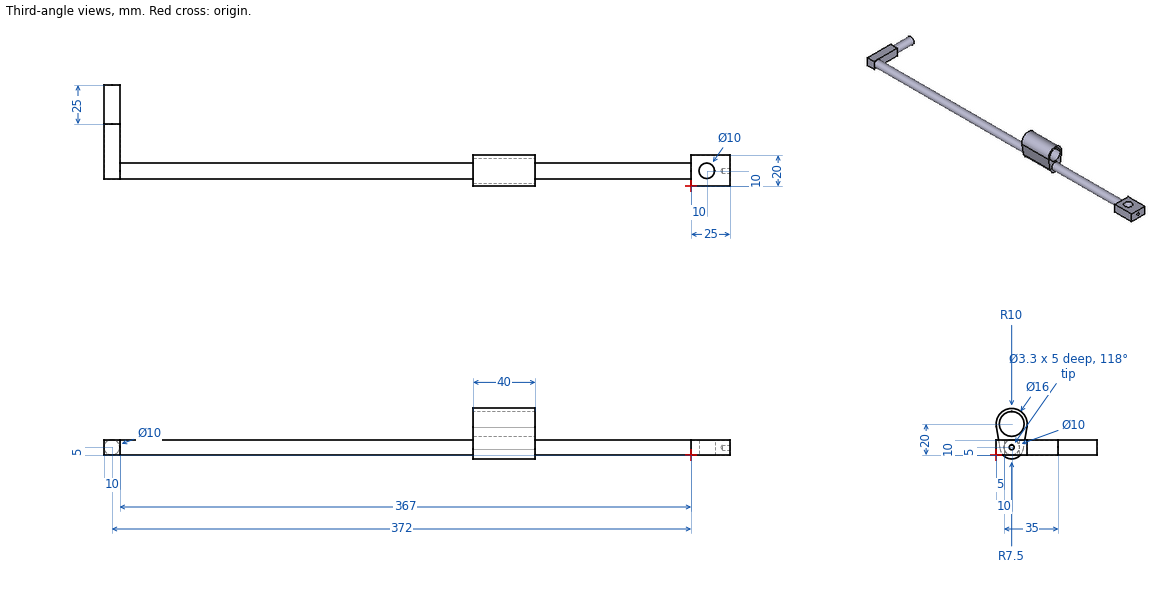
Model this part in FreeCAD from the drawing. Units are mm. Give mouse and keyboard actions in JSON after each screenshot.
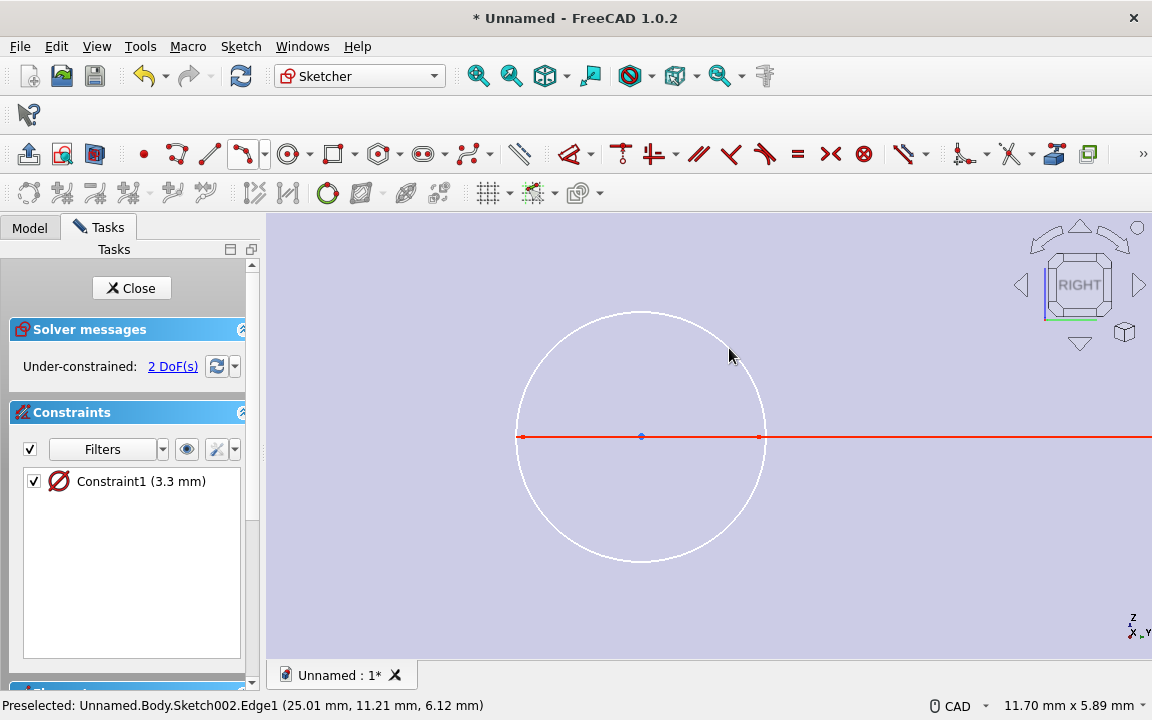
{"action": "key", "text": "d"}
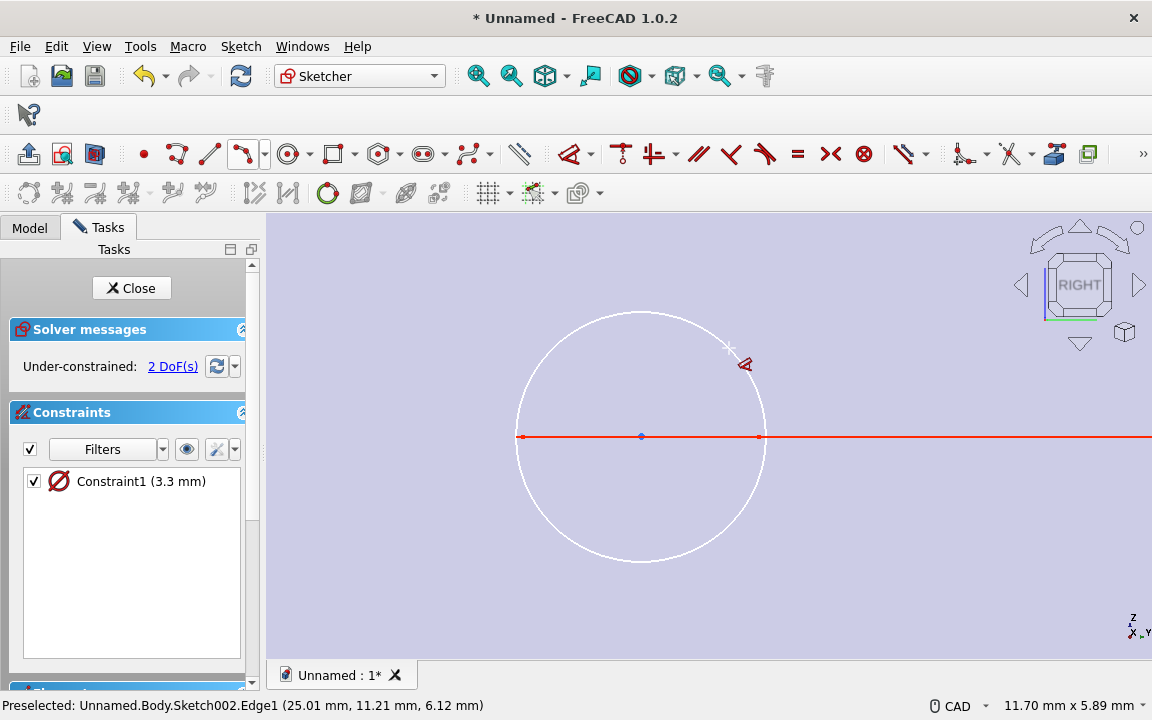
{"action": "left_click", "coordinate": [641, 437]}
{"action": "left_click", "coordinate": [675, 534]}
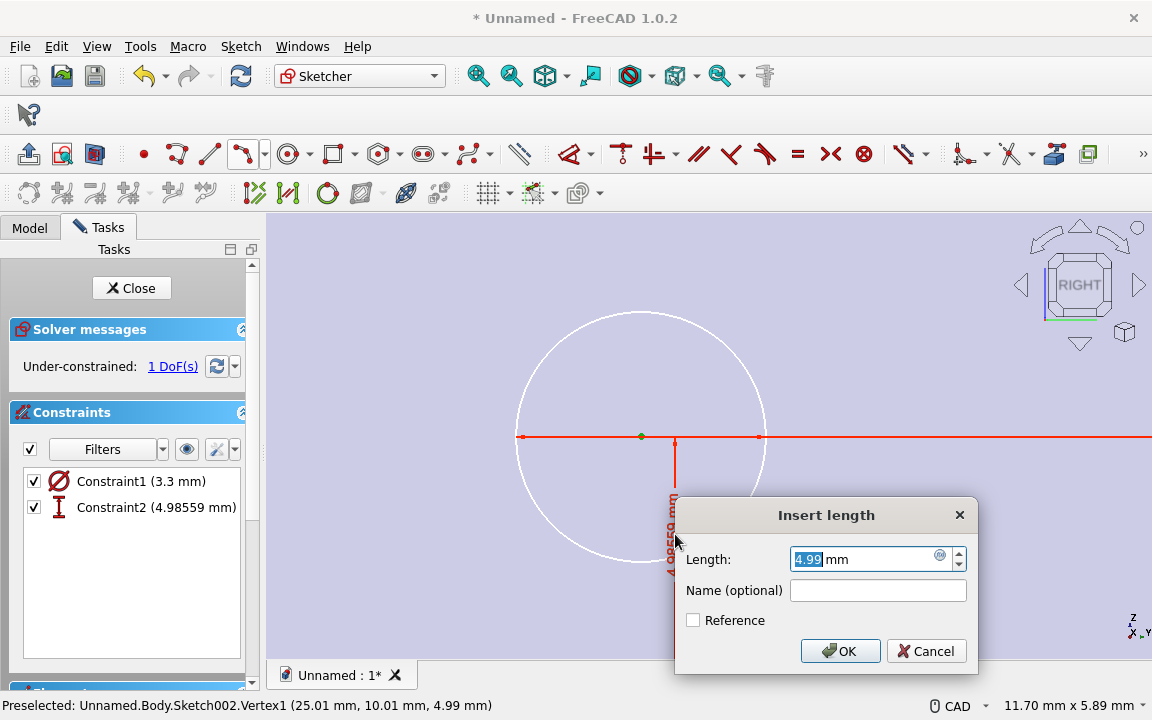
{"action": "type", "text": "5"}
{"action": "key", "text": "Return"}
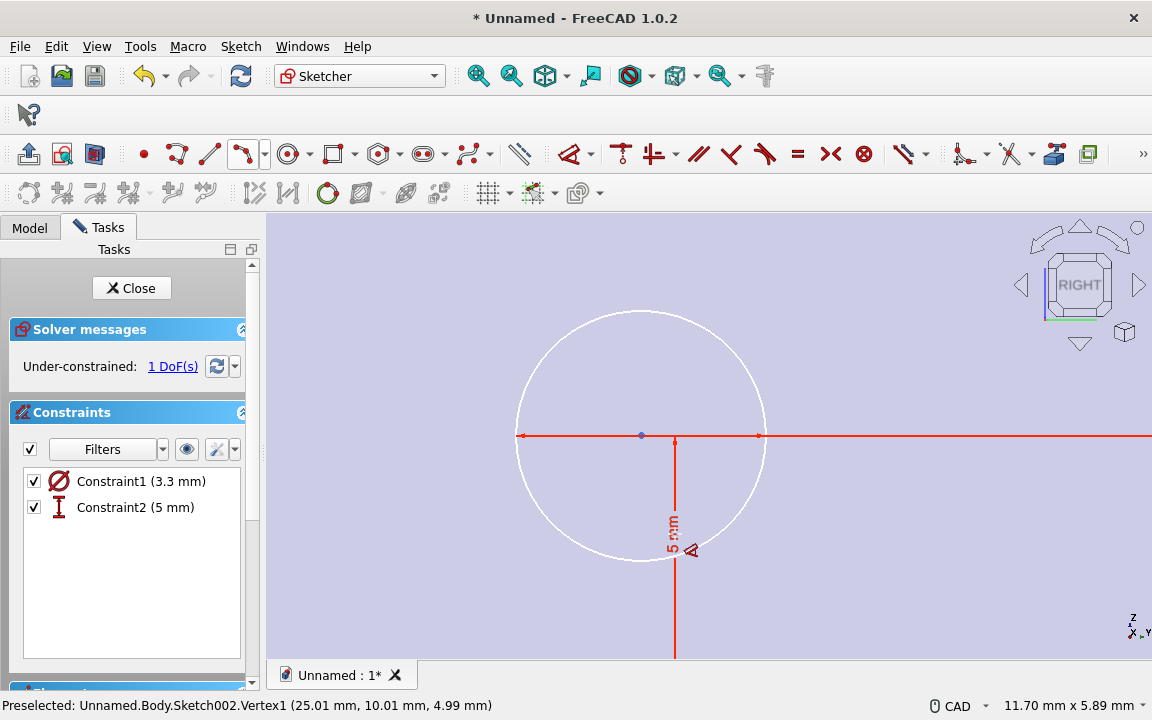
{"action": "left_click", "coordinate": [641, 436]}
{"action": "left_click", "coordinate": [467, 402]}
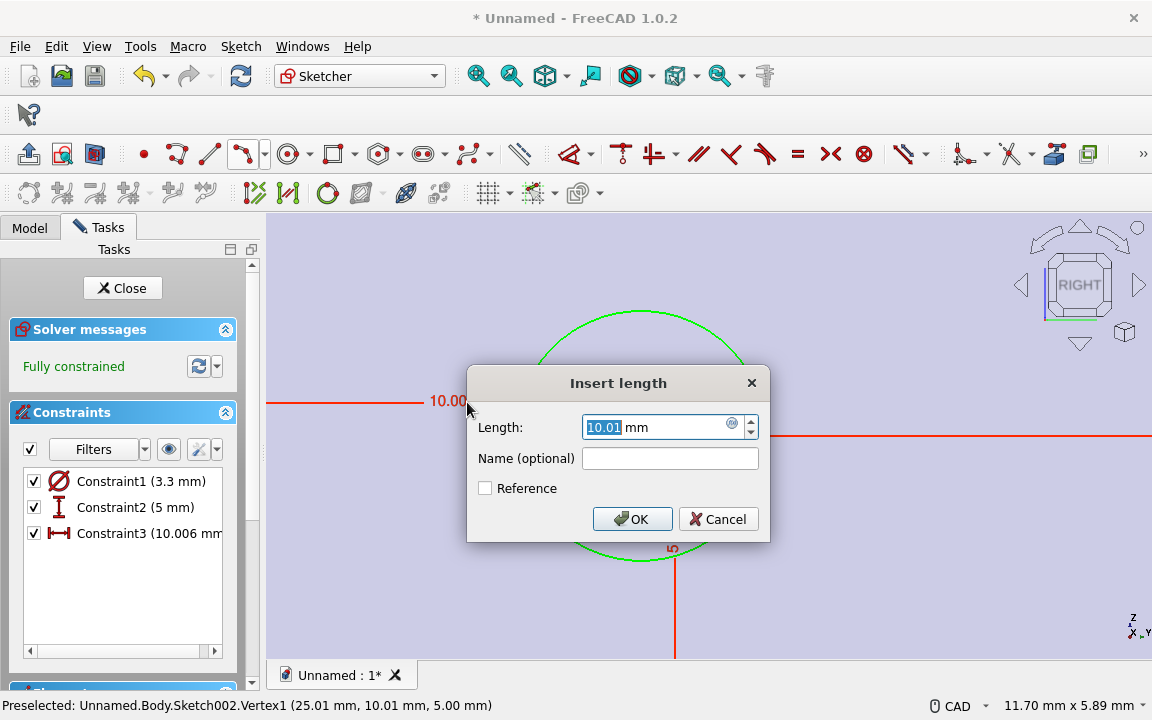
{"action": "type", "text": "10"}
{"action": "key", "text": "Return"}
{"action": "key", "text": "Escape"}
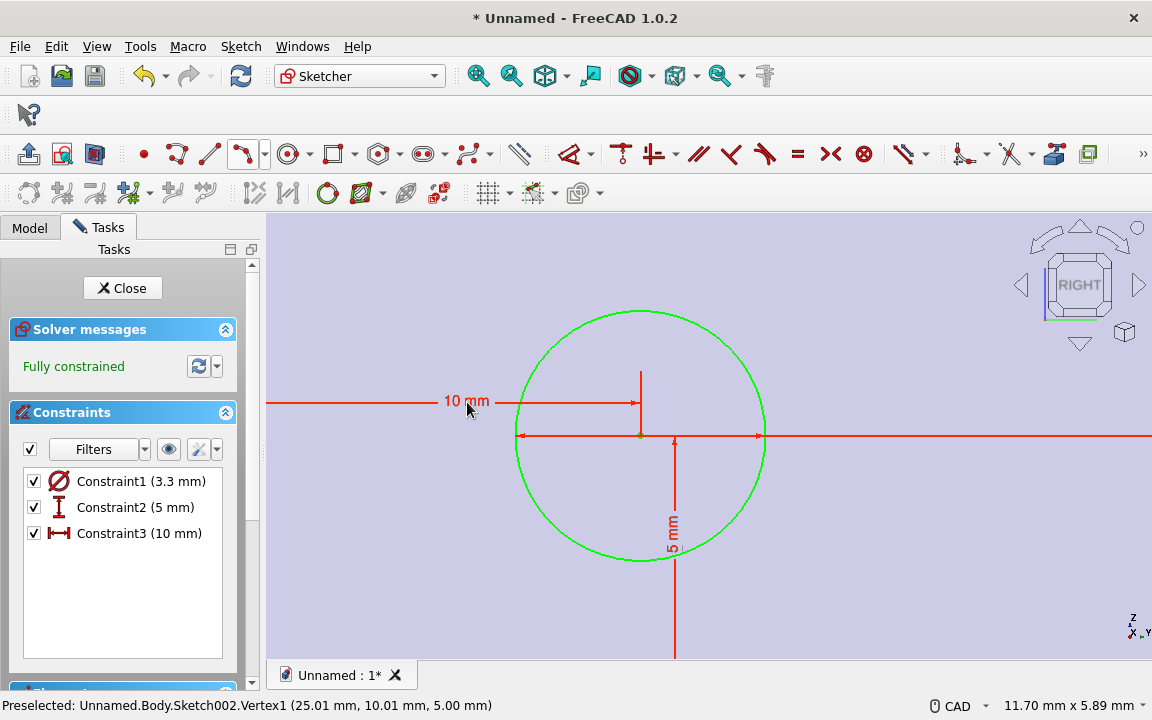
{"action": "left_click", "coordinate": [123, 288]}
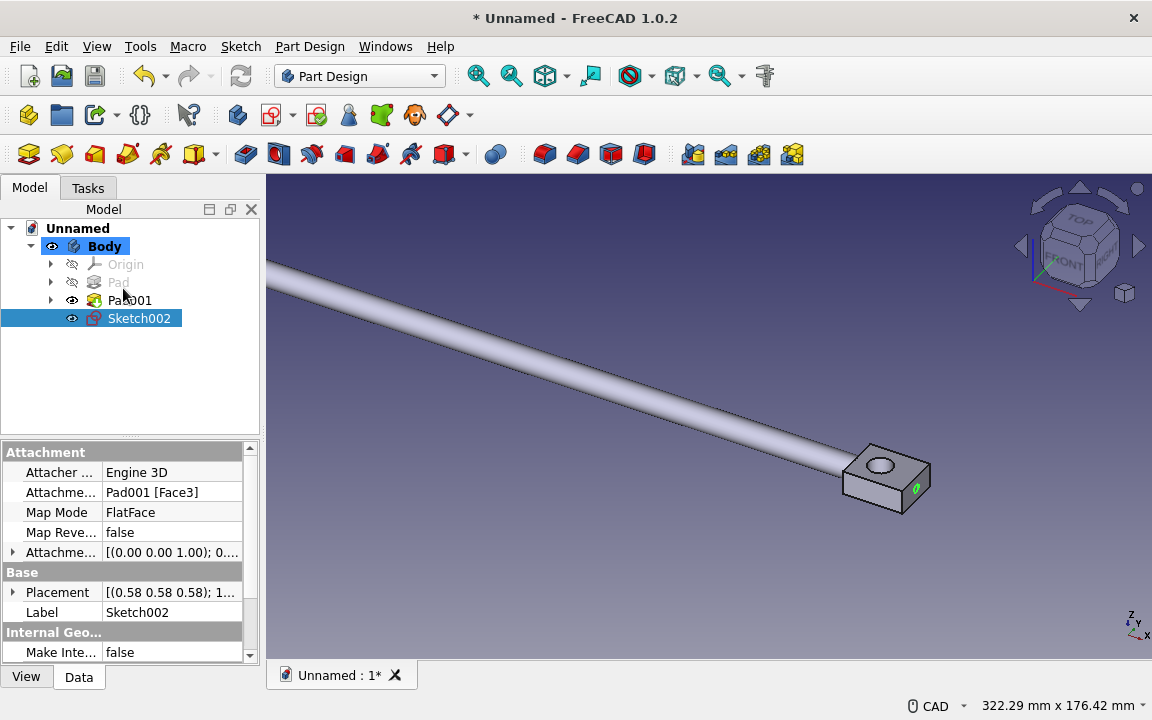
{"action": "left_click", "coordinate": [279, 154]}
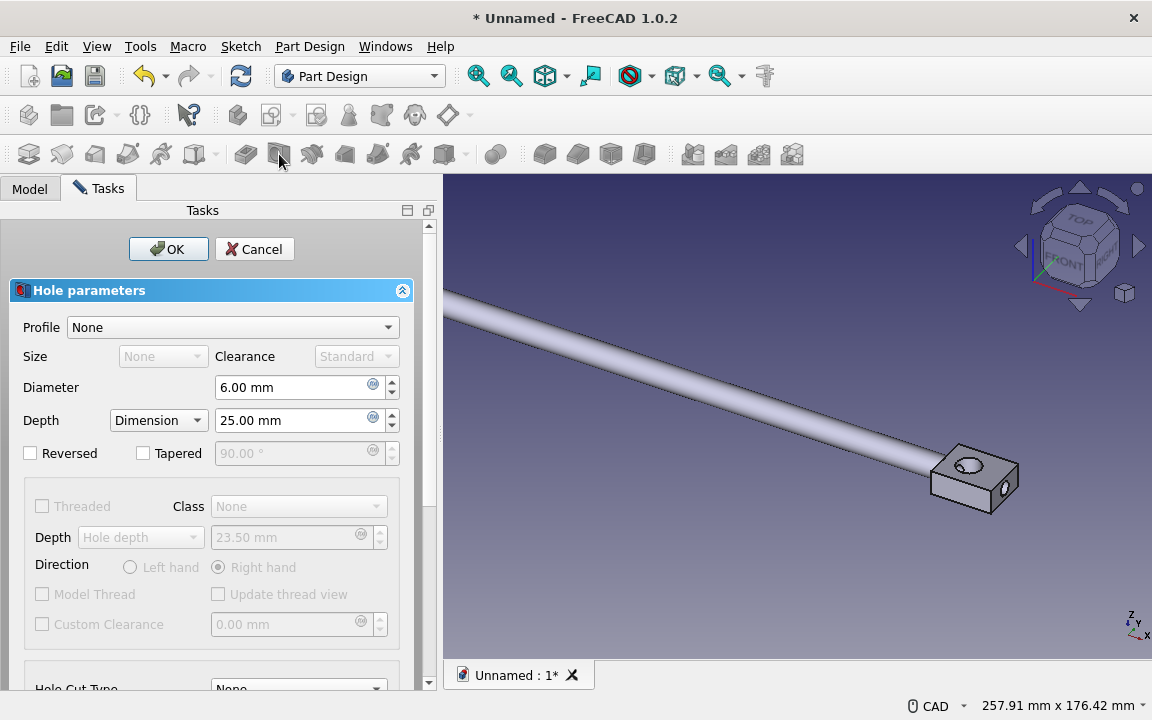
{"action": "triple_click", "coordinate": [300, 388]}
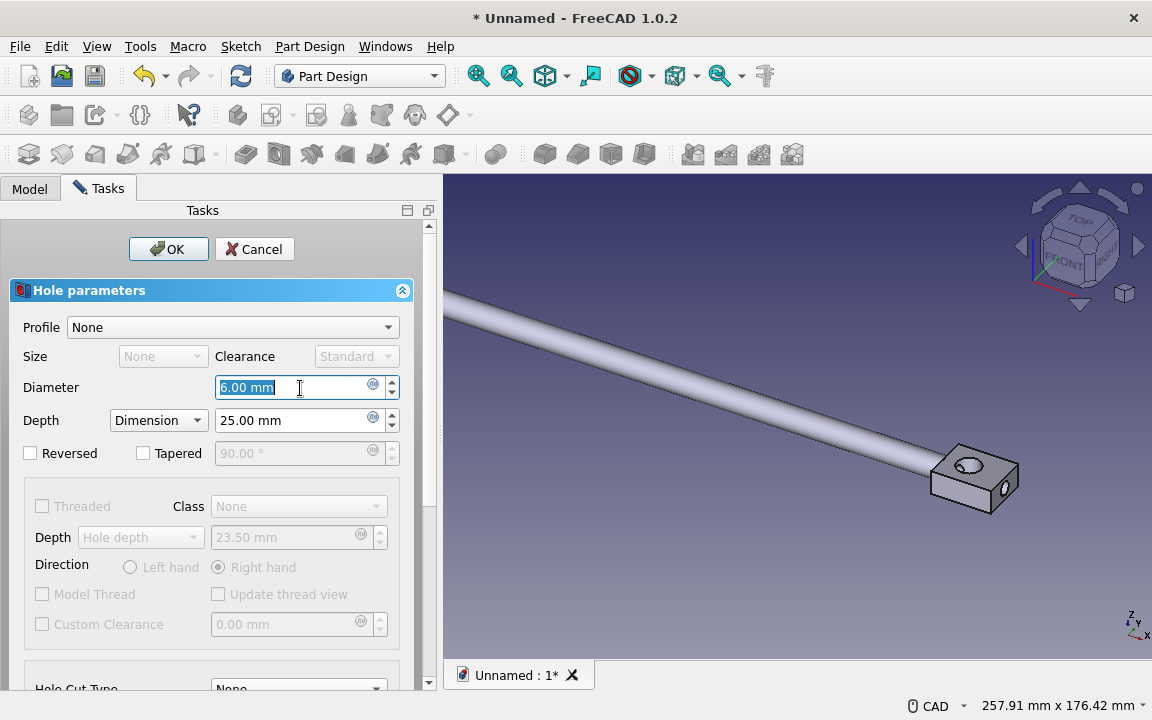
{"action": "type", "text": "3.3"}
{"action": "key", "text": "Tab"}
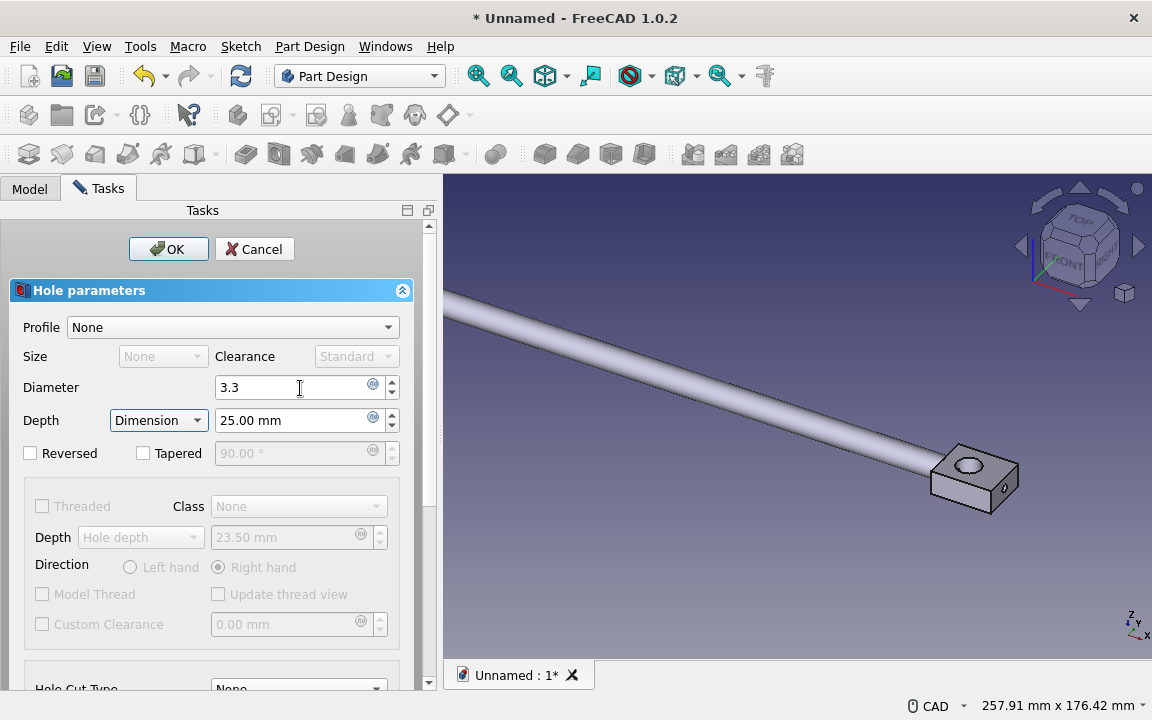
{"action": "triple_click", "coordinate": [300, 420]}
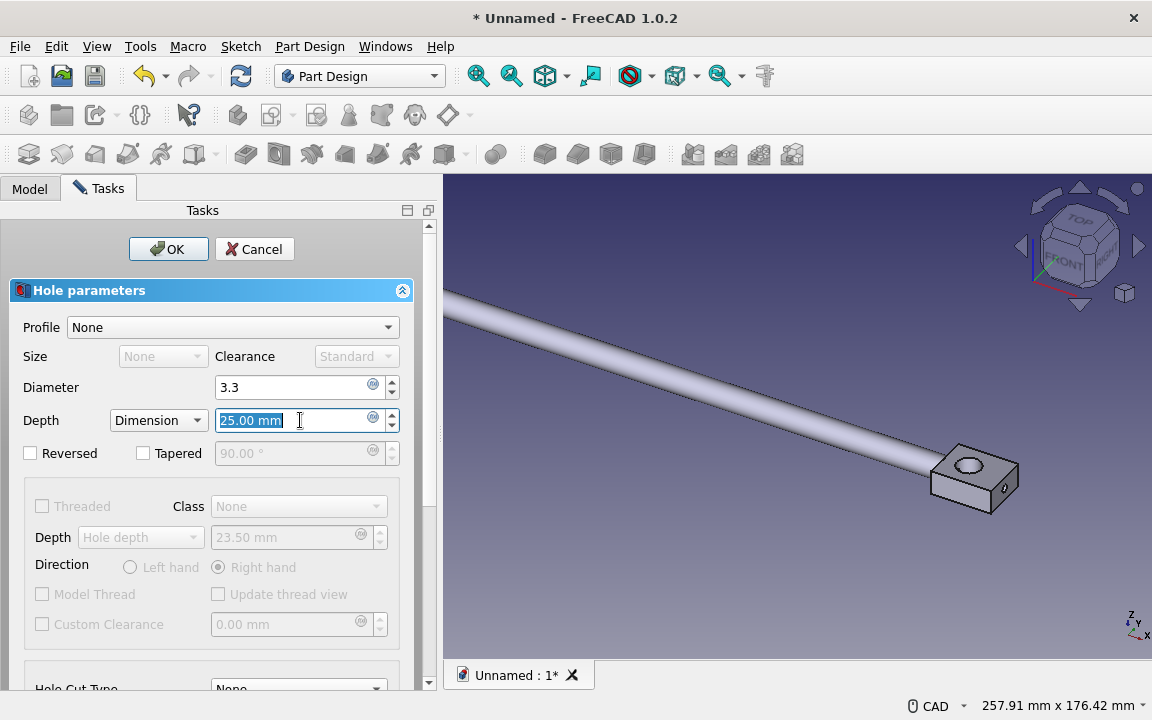
{"action": "type", "text": "5"}
{"action": "key", "text": "Tab"}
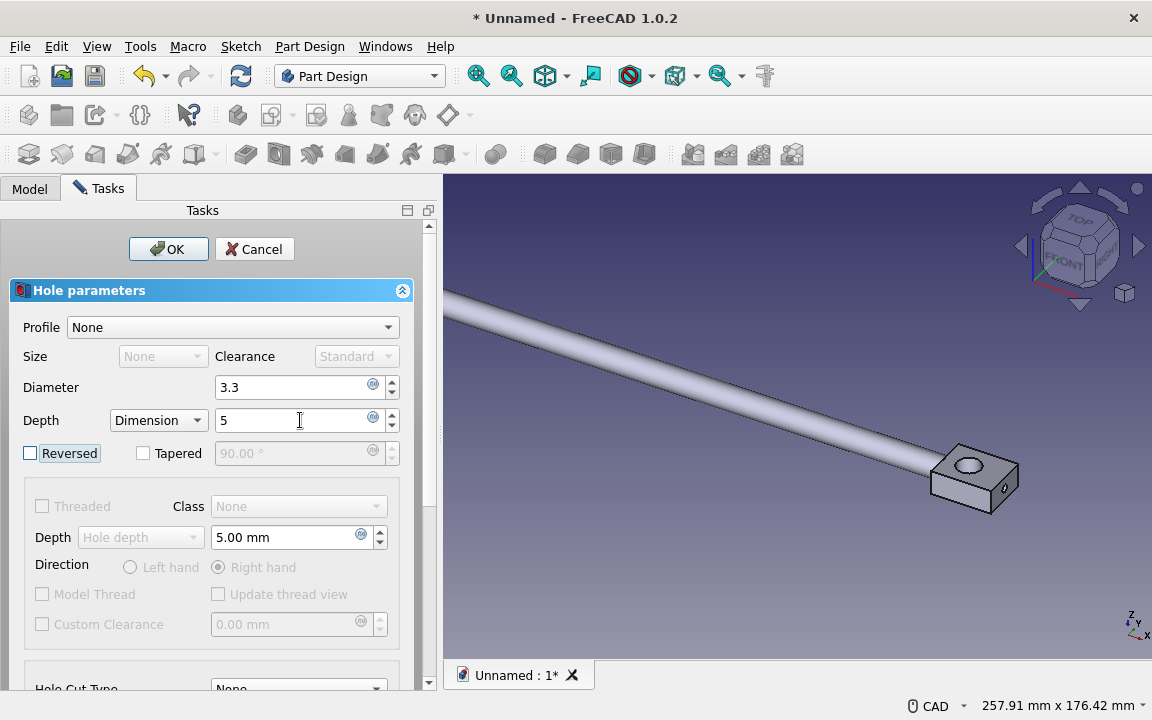
{"action": "left_click", "coordinate": [169, 249]}